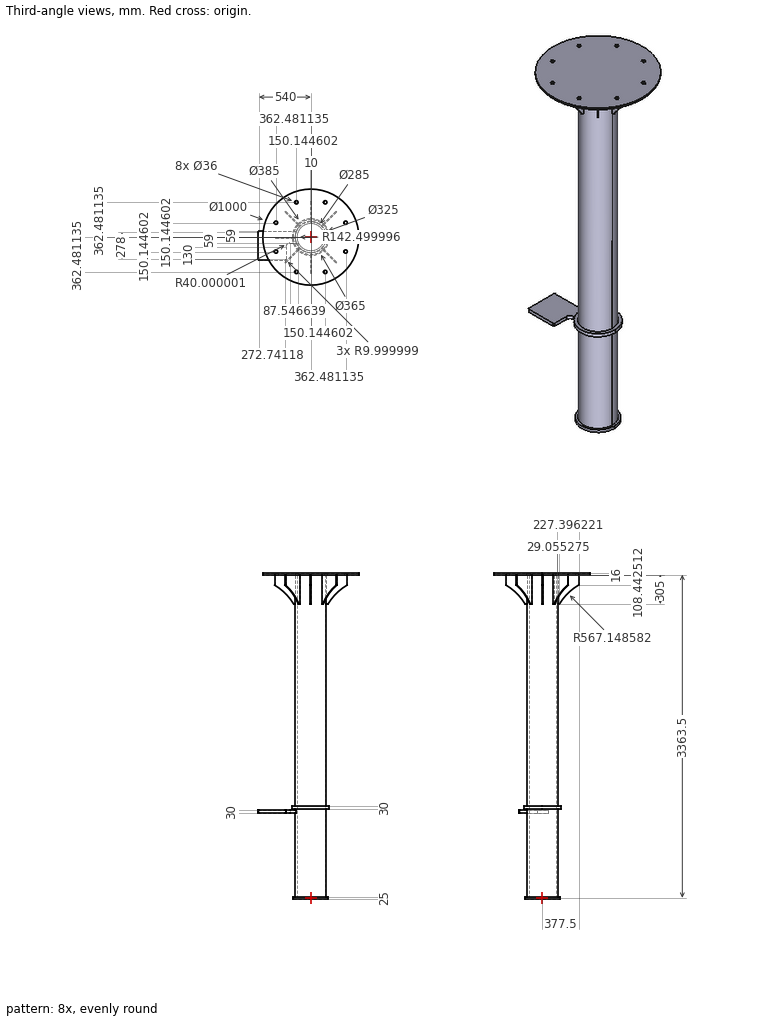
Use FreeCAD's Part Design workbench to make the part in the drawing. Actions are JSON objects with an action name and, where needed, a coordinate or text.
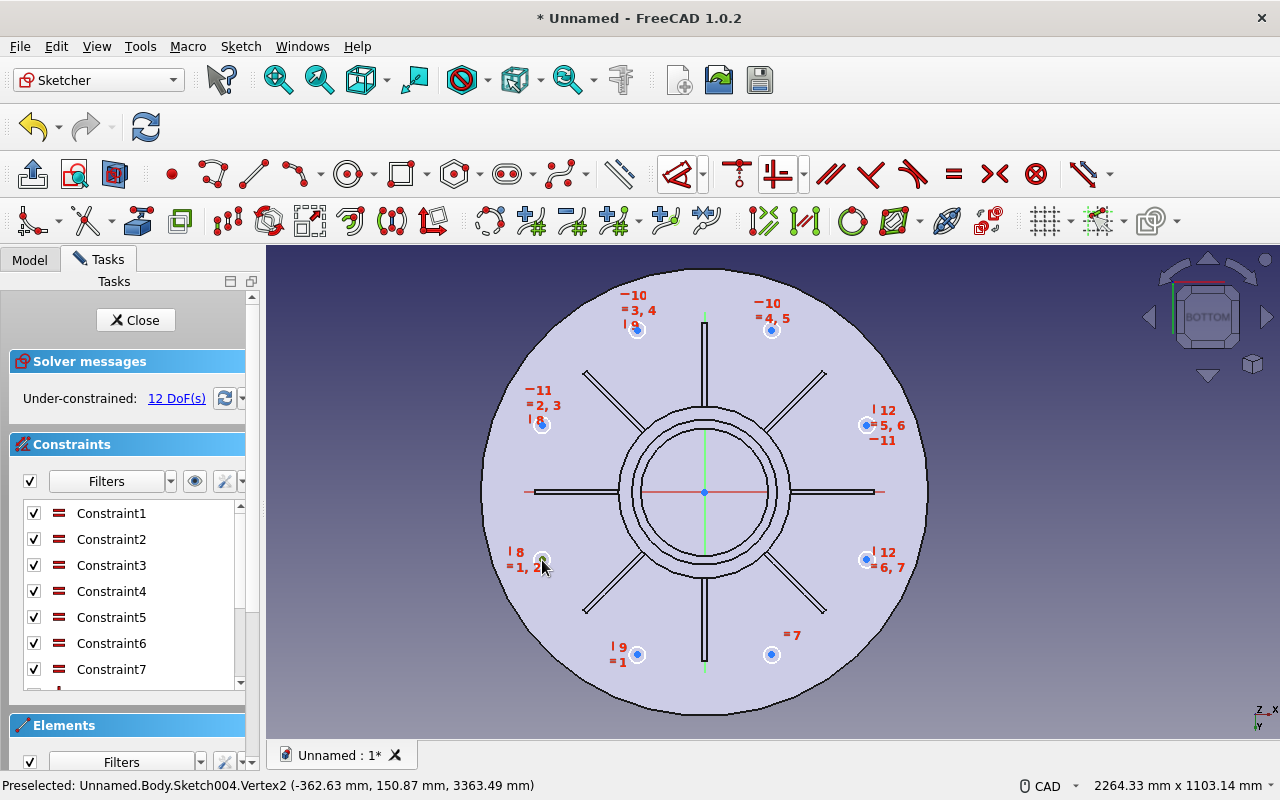
{"action": "left_click", "coordinate": [867, 560]}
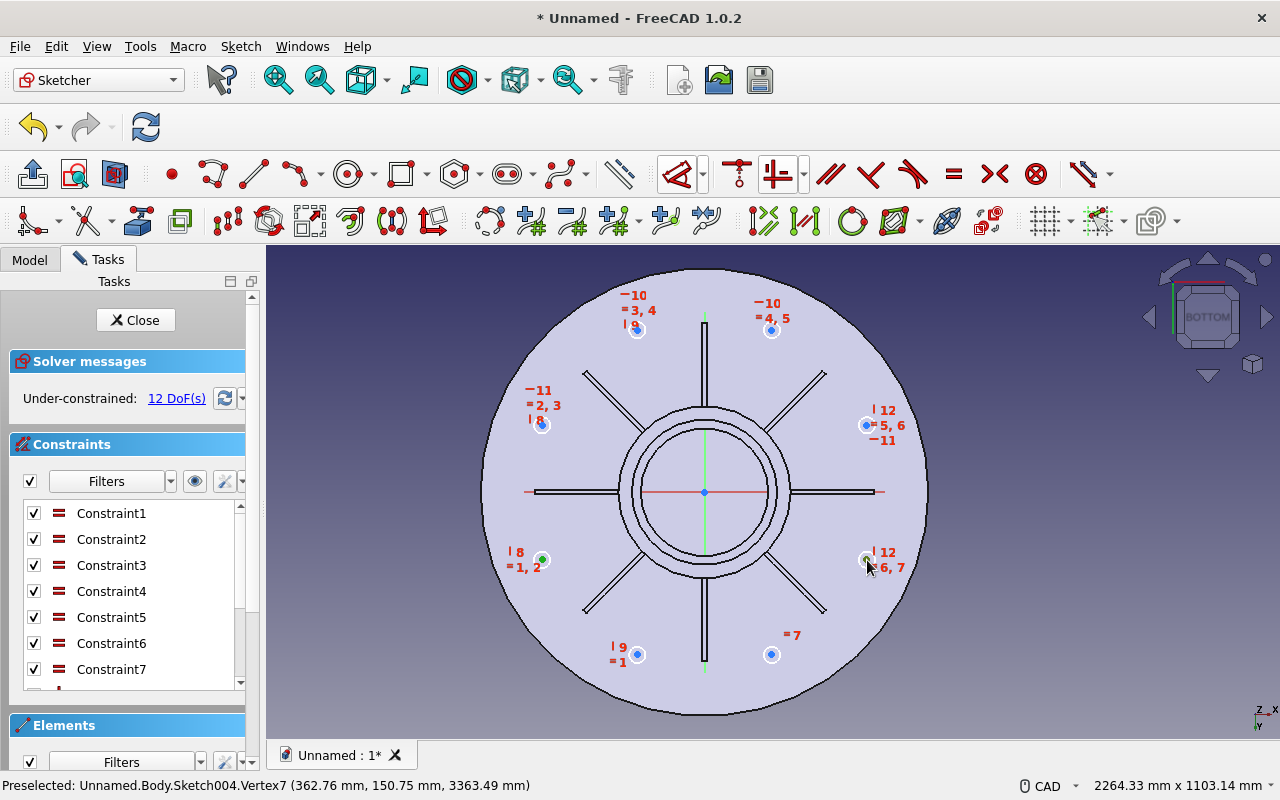
{"action": "key", "text": "h"}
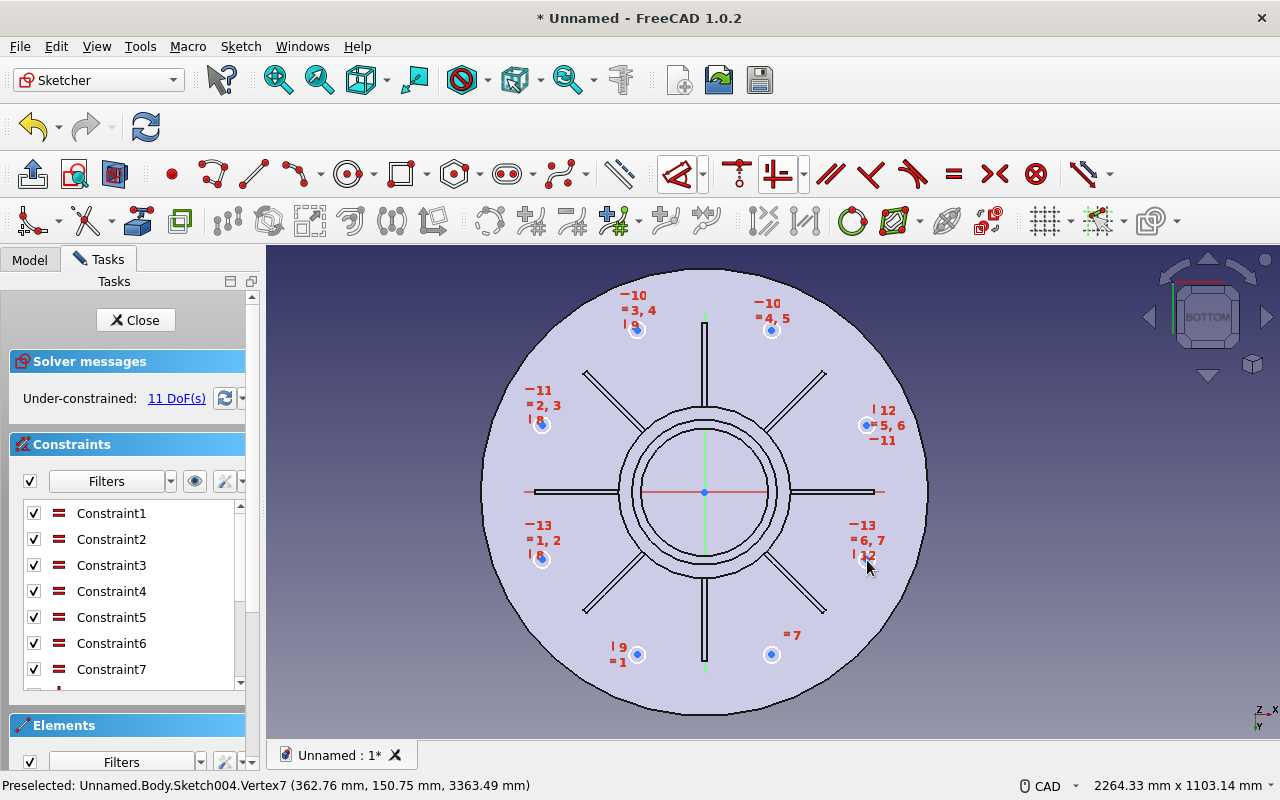
{"action": "left_click", "coordinate": [772, 330]}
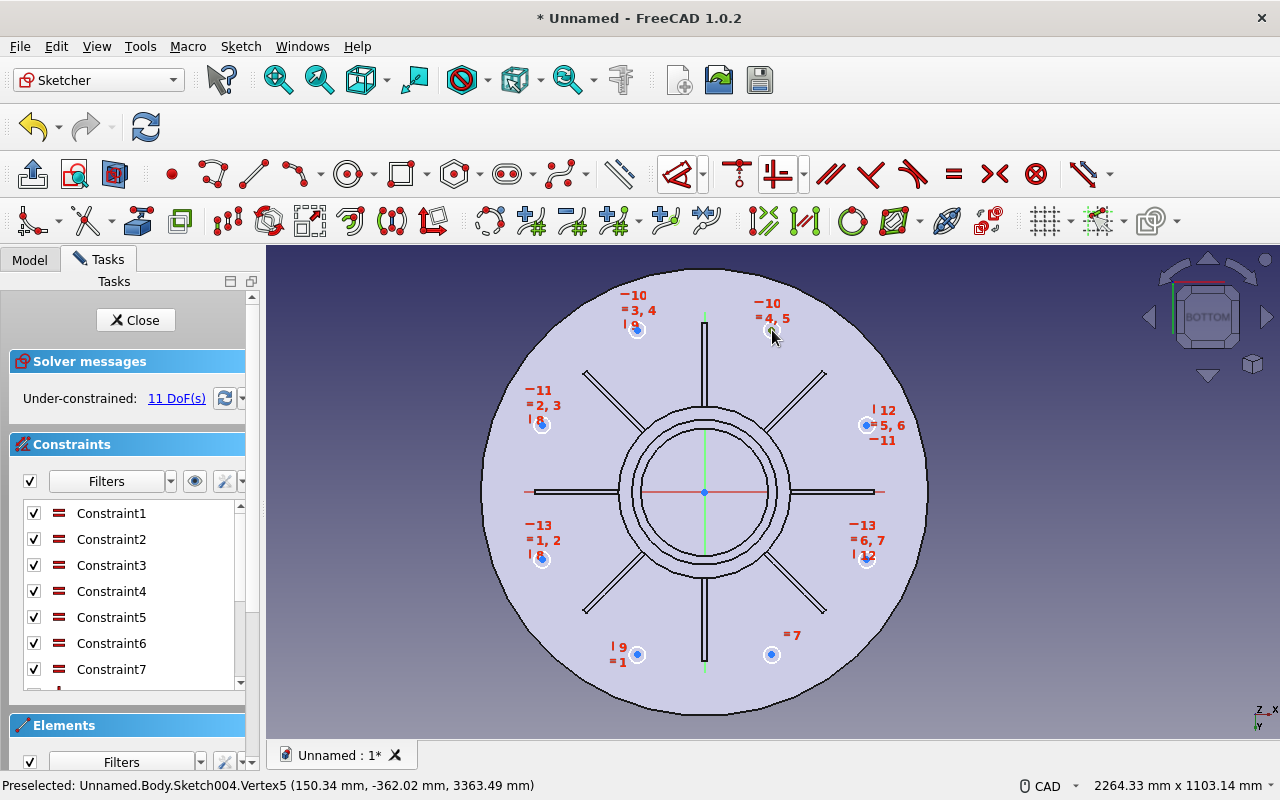
{"action": "left_click", "coordinate": [772, 655]}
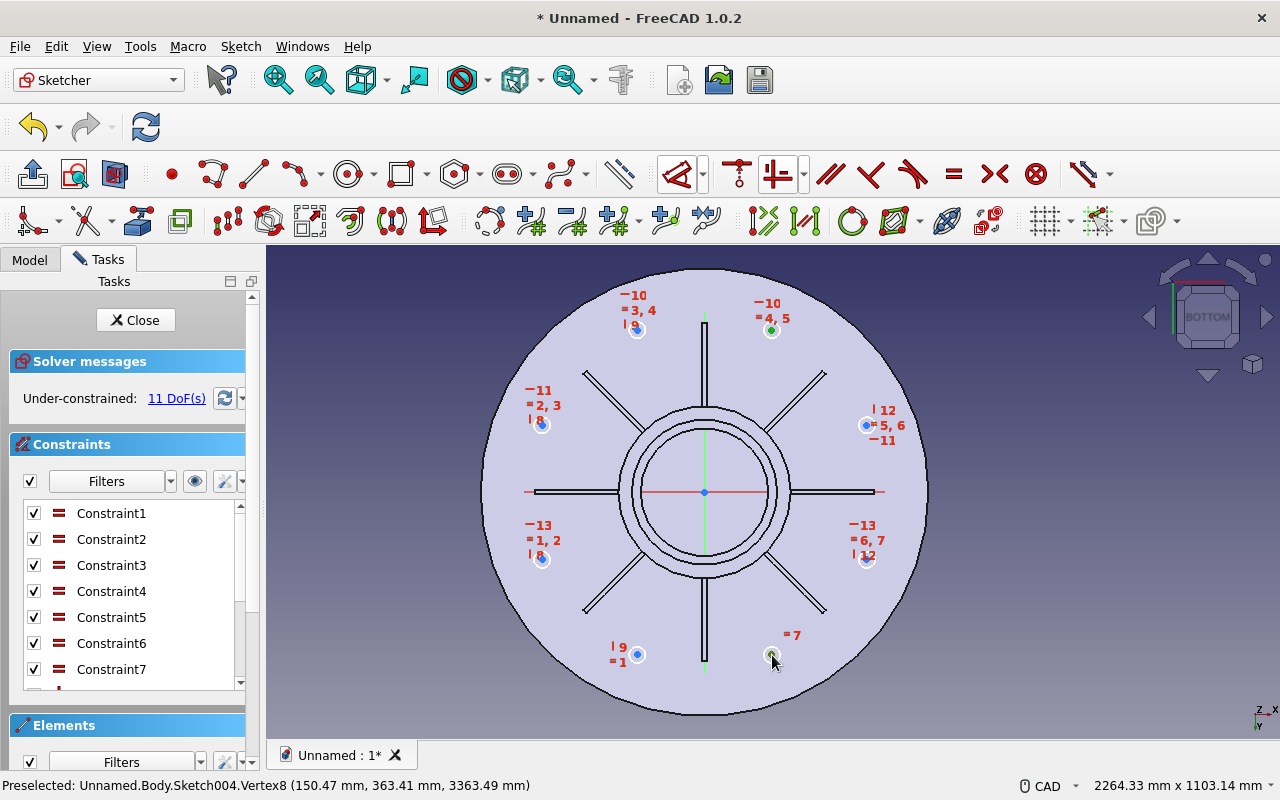
{"action": "key", "text": "v"}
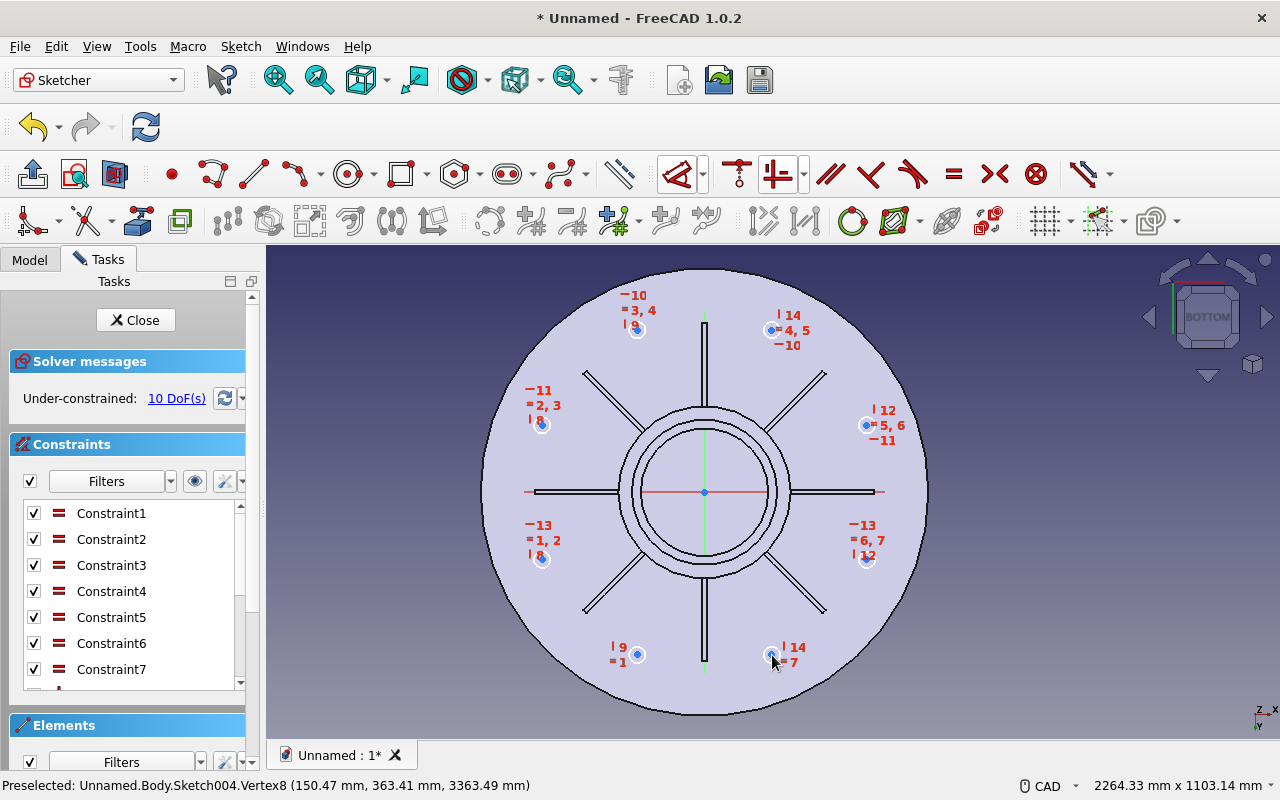
{"action": "left_click", "coordinate": [637, 655]}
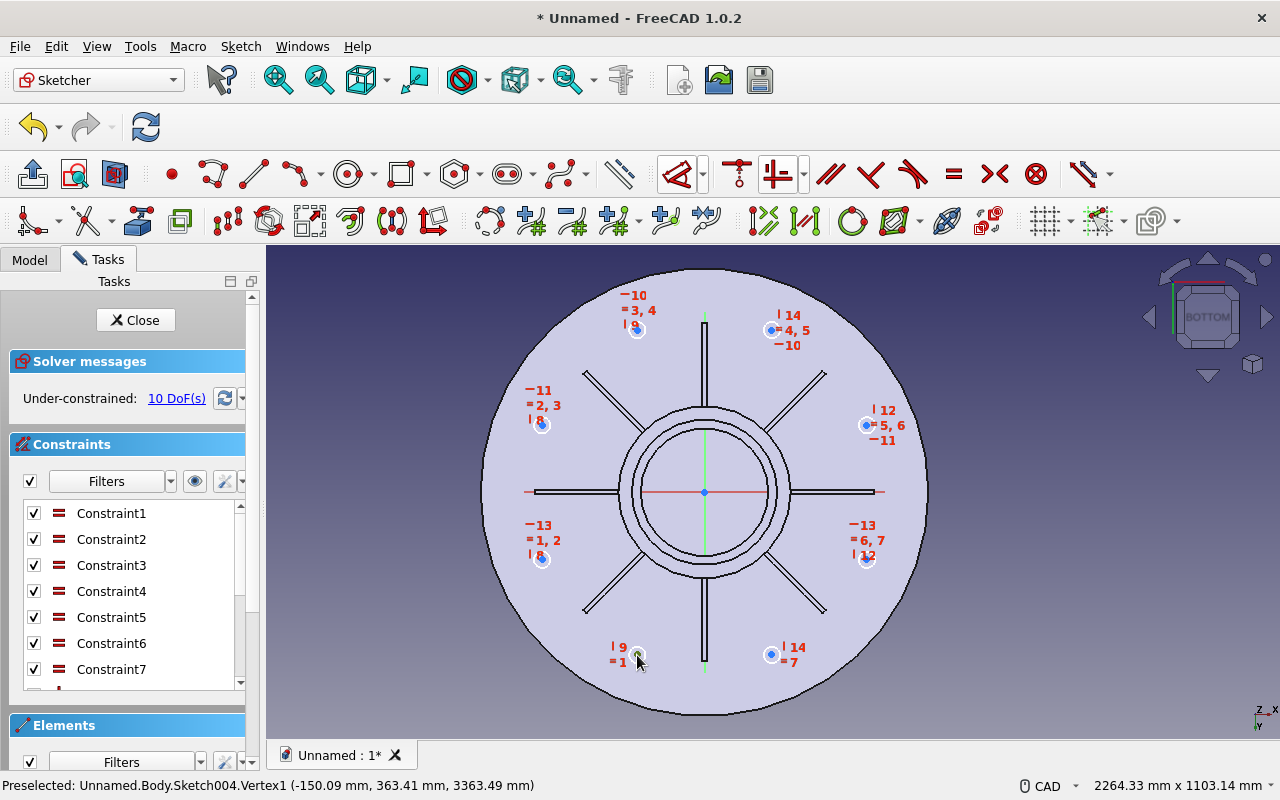
{"action": "left_click", "coordinate": [772, 655]}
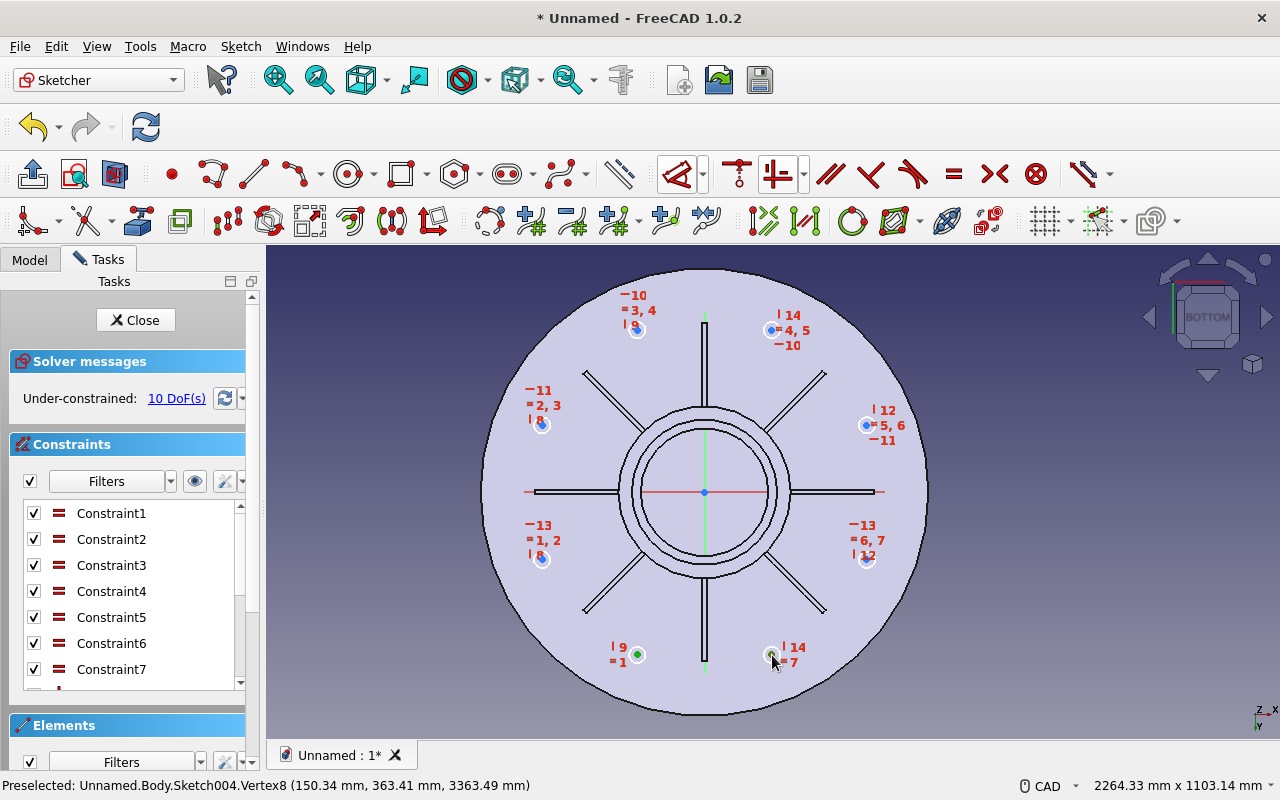
{"action": "key", "text": "h"}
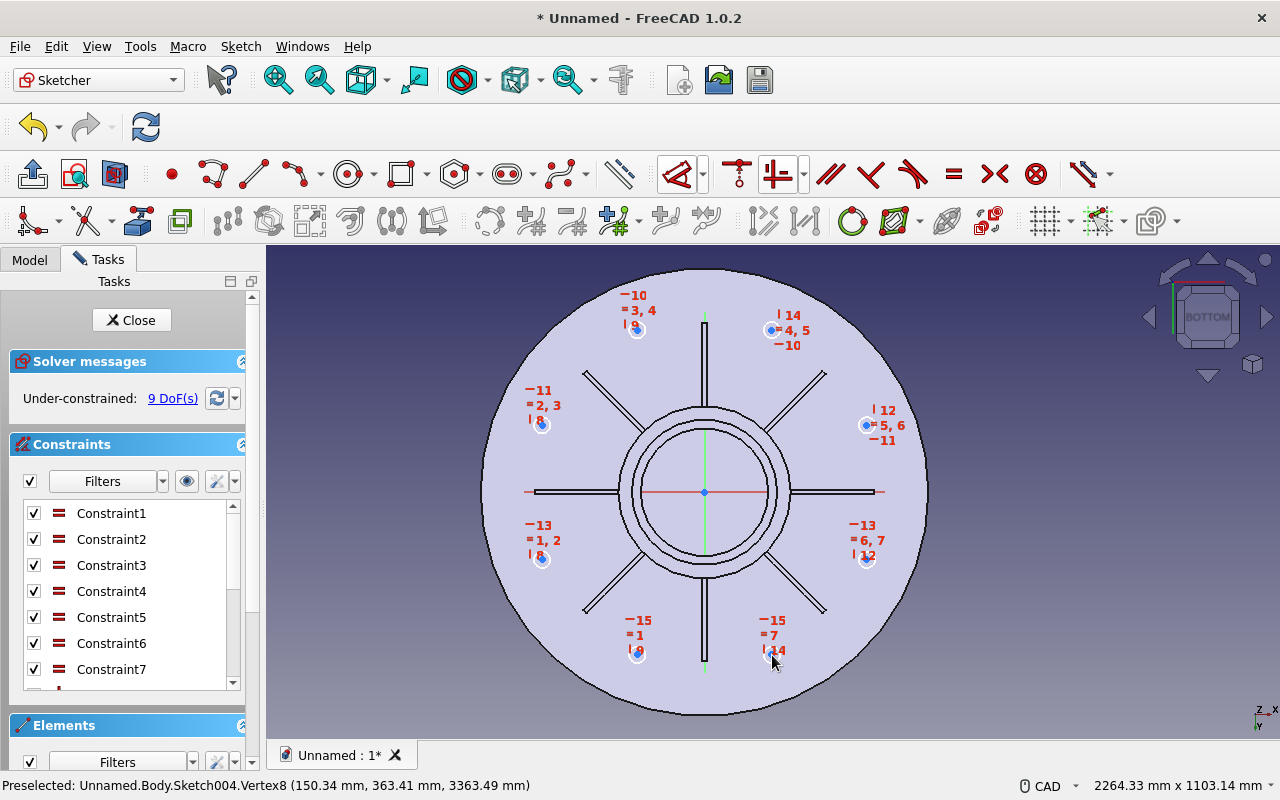
{"action": "scroll", "coordinate": [632, 649], "scroll_direction": "up", "scroll_amount": 5}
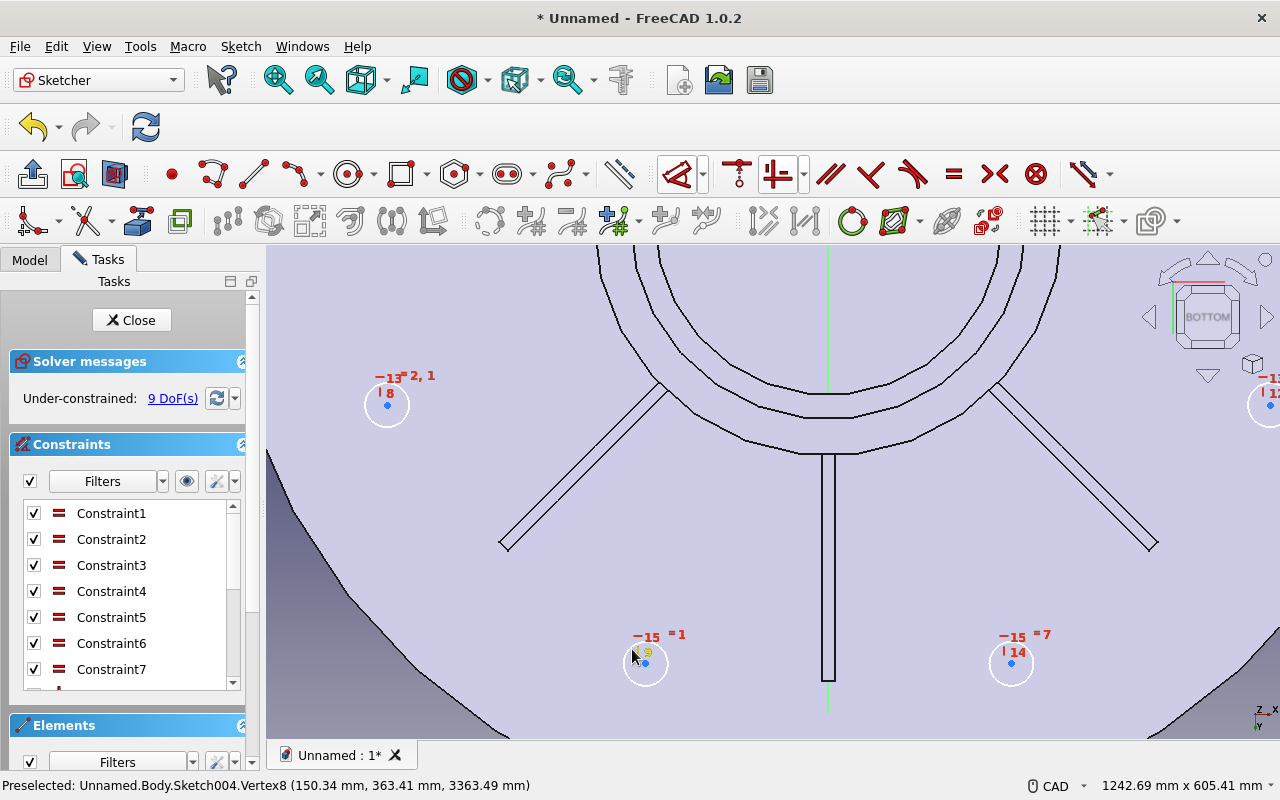
{"action": "left_click", "coordinate": [630, 648]}